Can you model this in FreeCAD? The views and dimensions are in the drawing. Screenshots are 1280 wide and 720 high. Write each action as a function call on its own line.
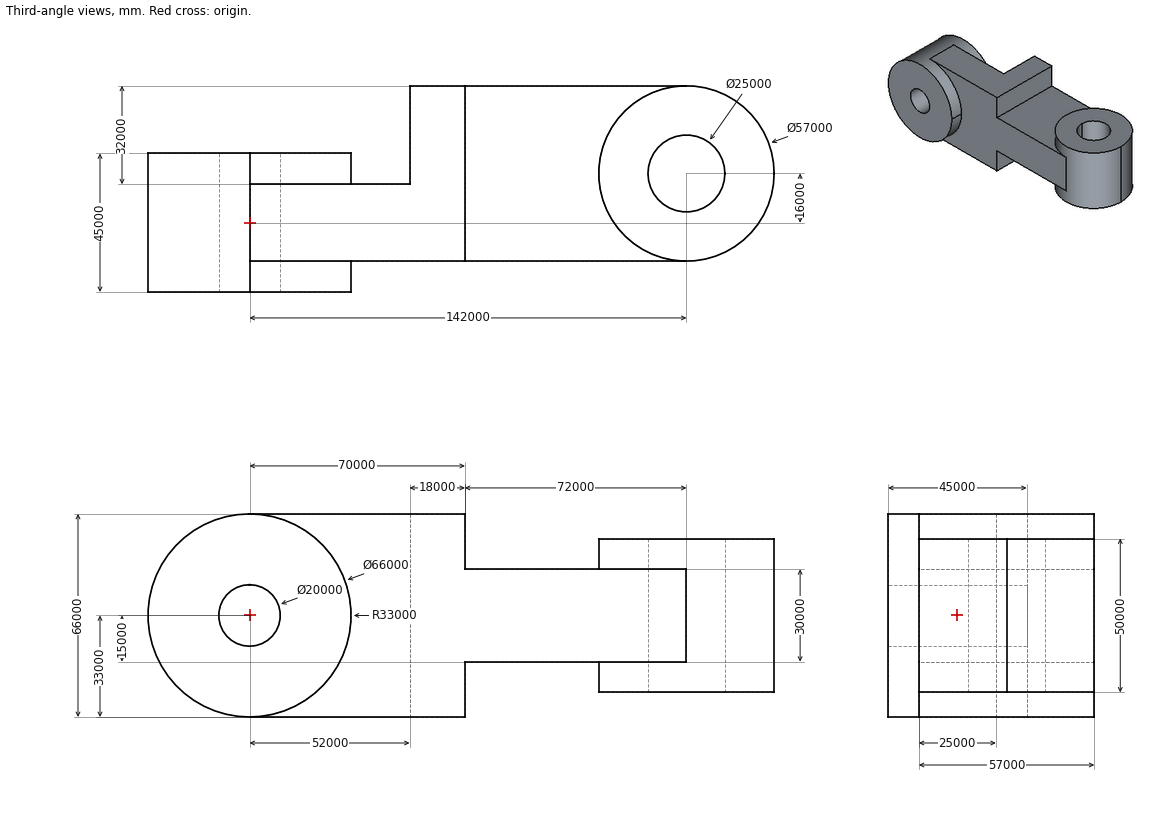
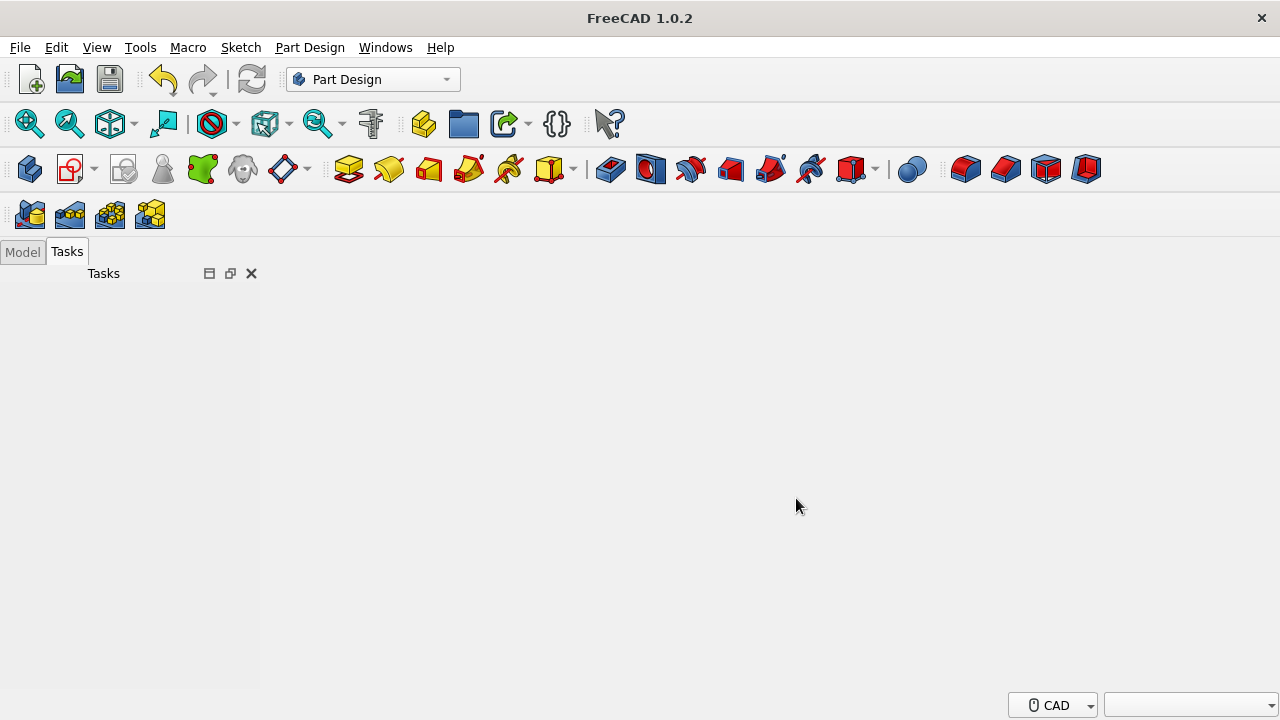
key(ctrl+n)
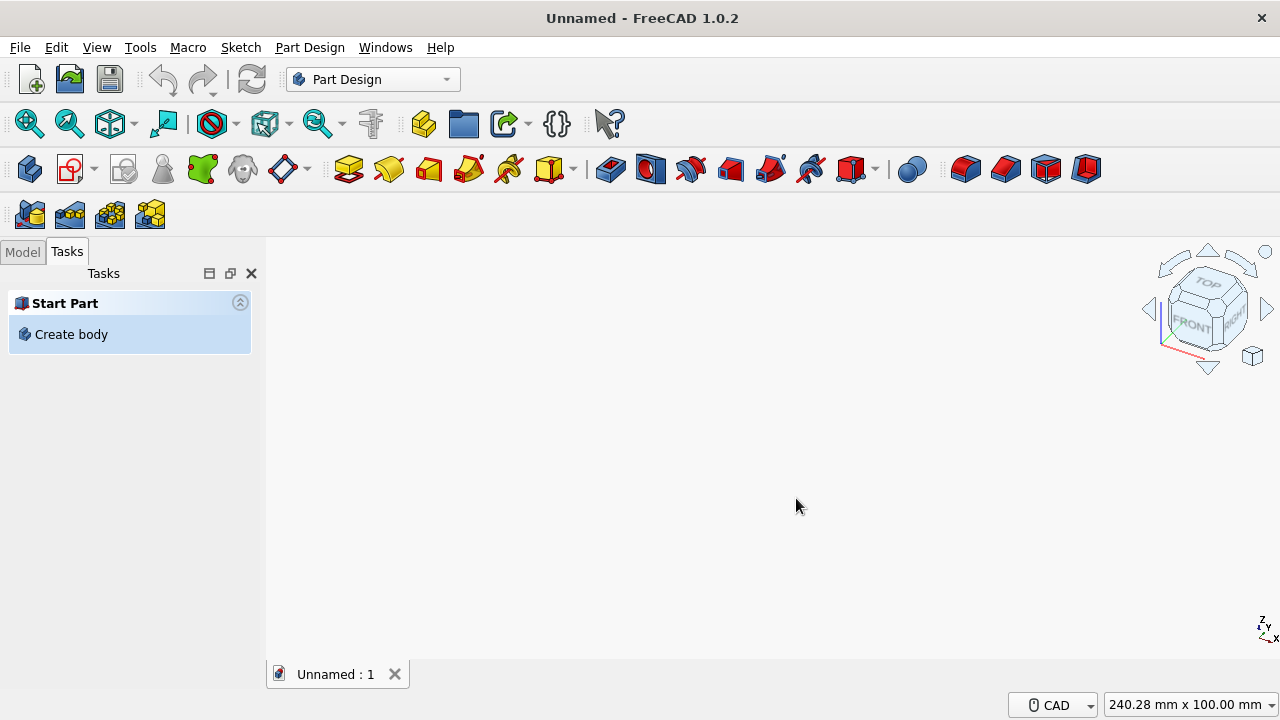
click(70, 170)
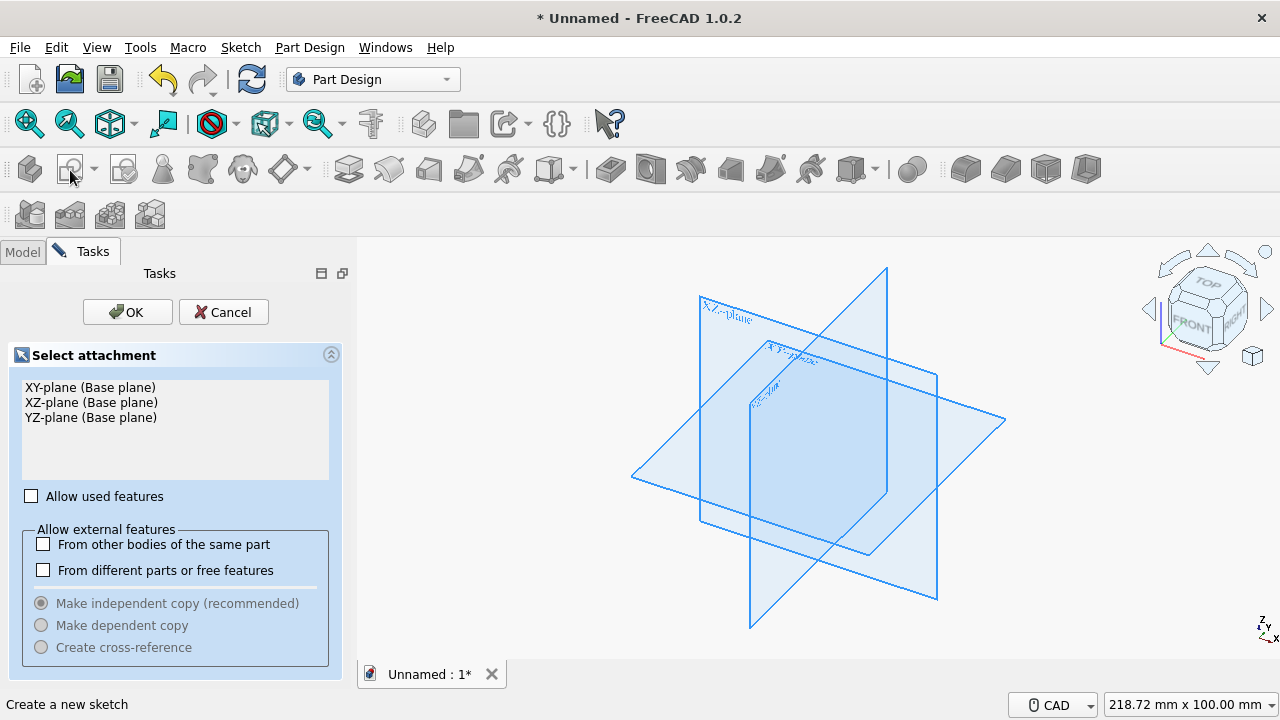
click(82, 402)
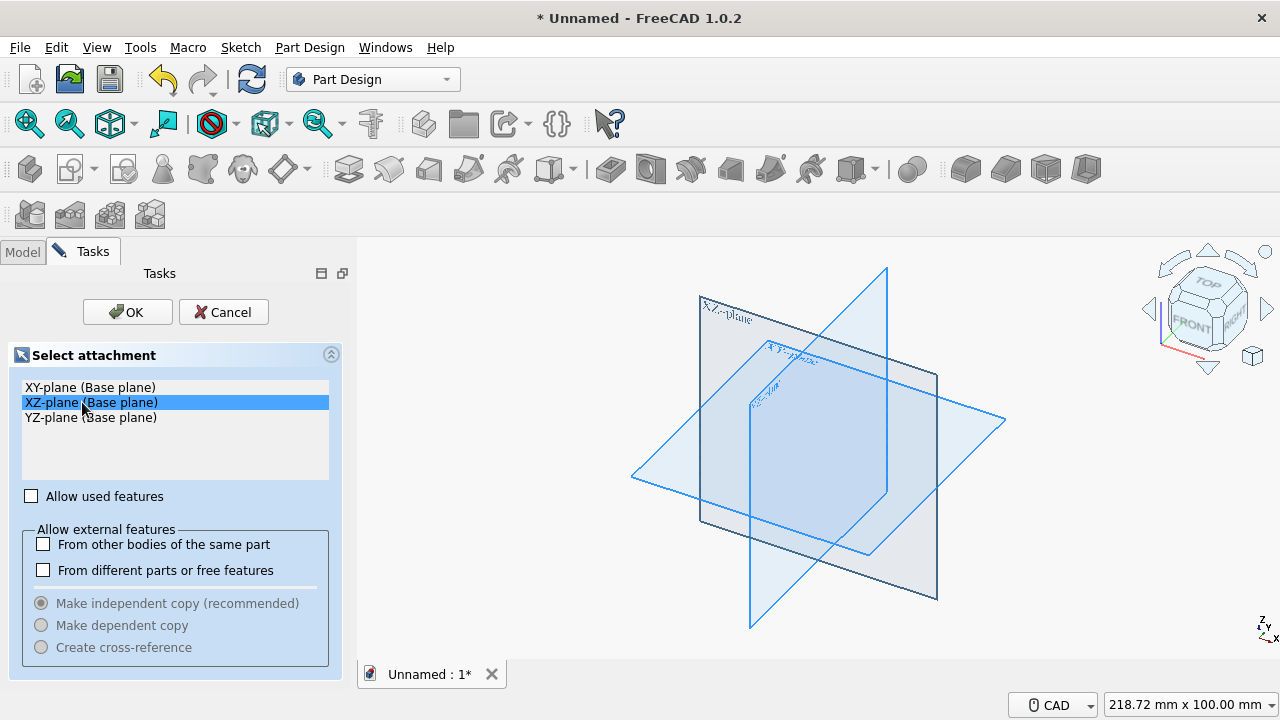
click(128, 312)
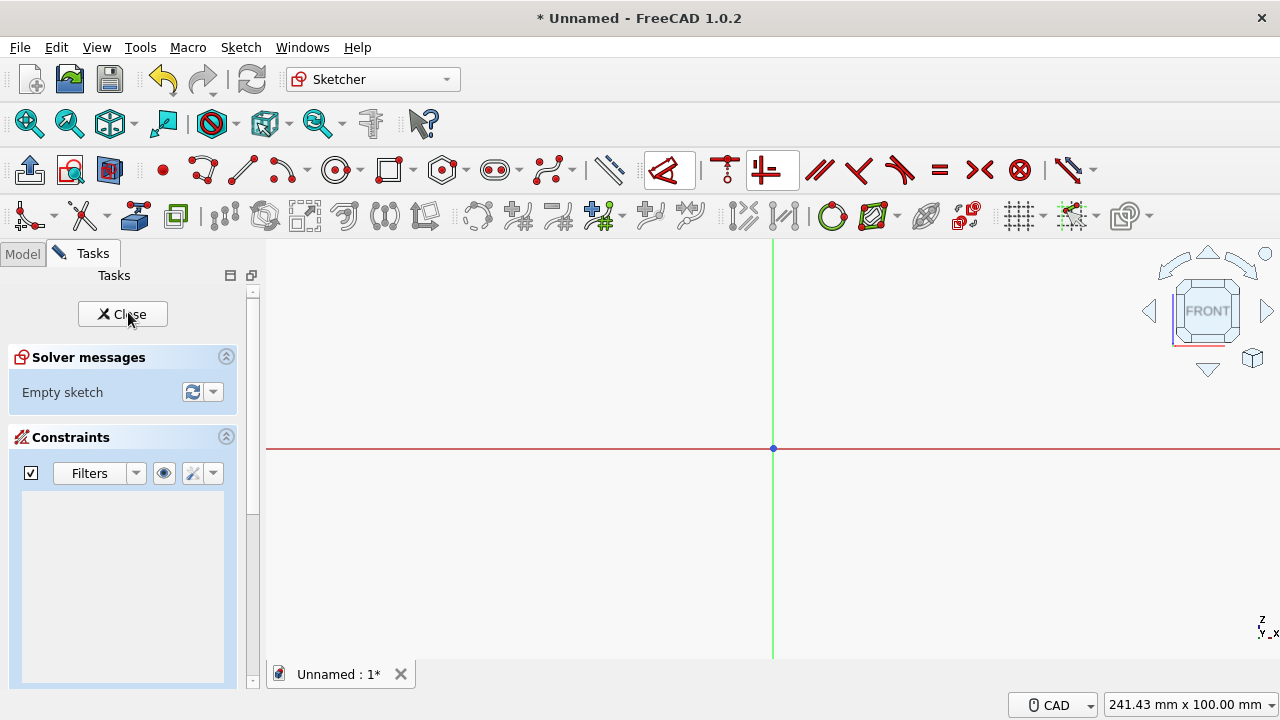
scroll(704, 449, down, 15)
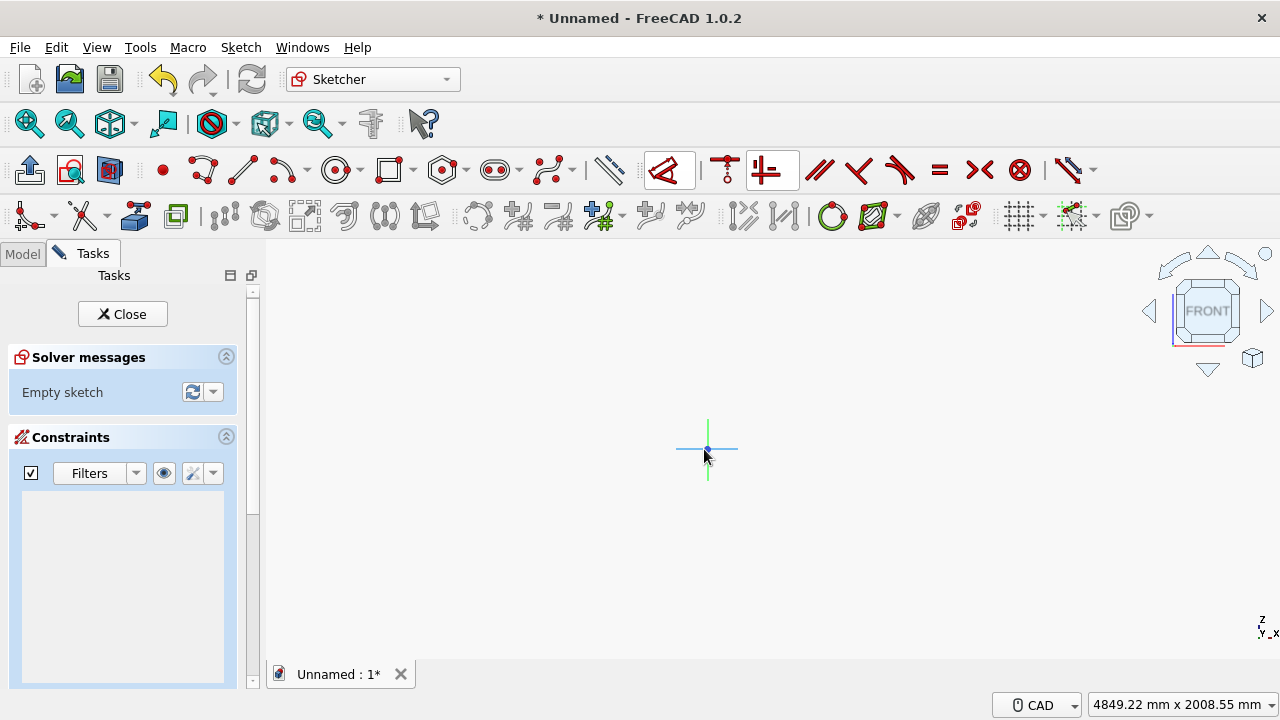
scroll(704, 449, down, 15)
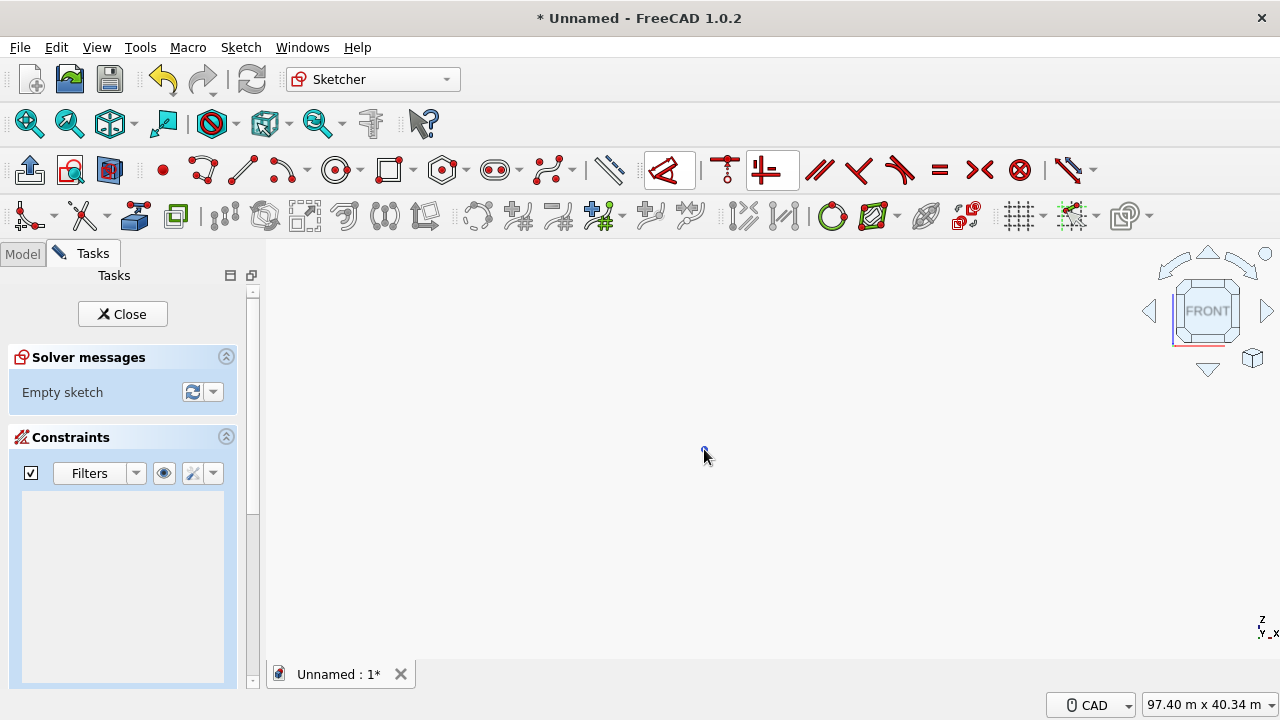
scroll(704, 449, down, 5)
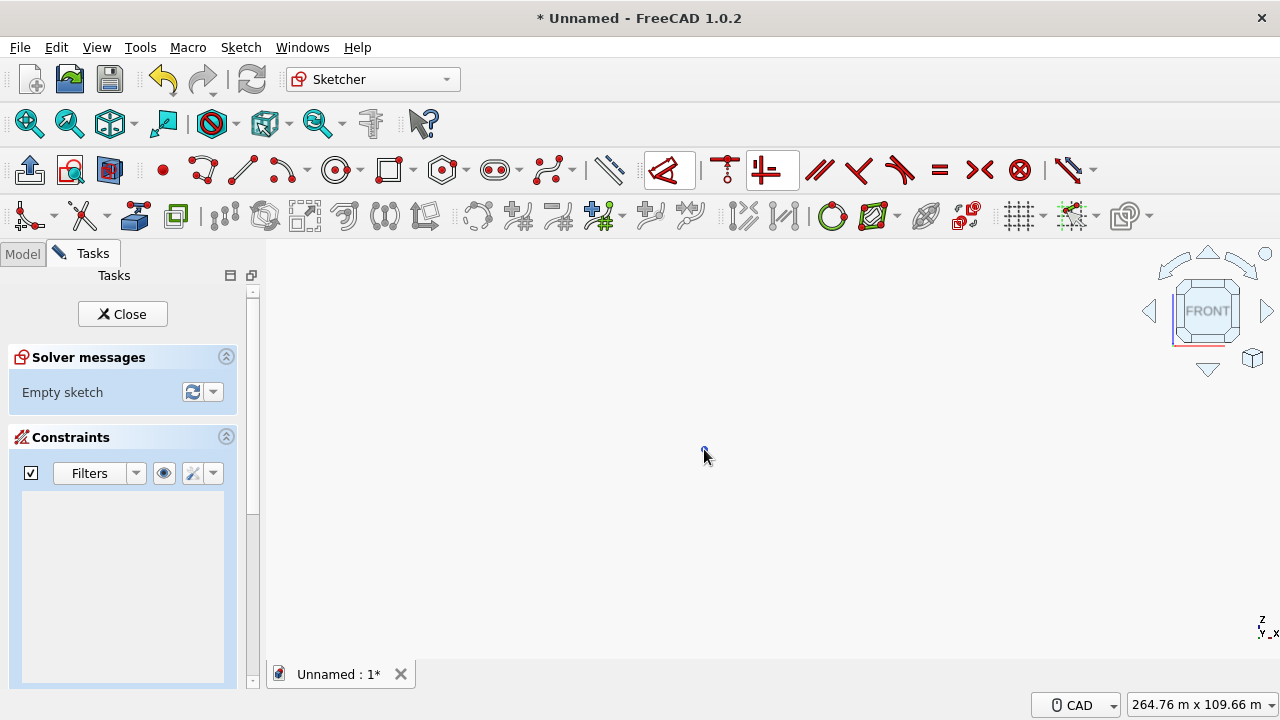
key(g)
key(c)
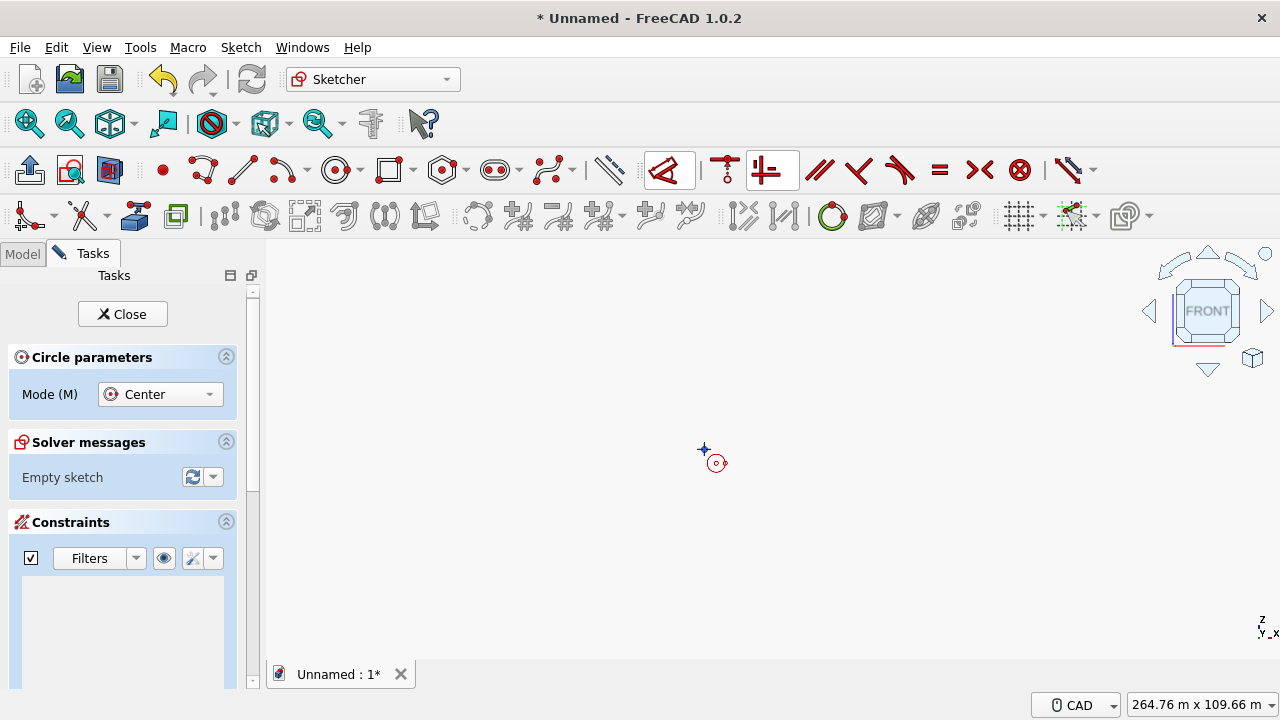
click(704, 450)
click(794, 360)
key(Escape)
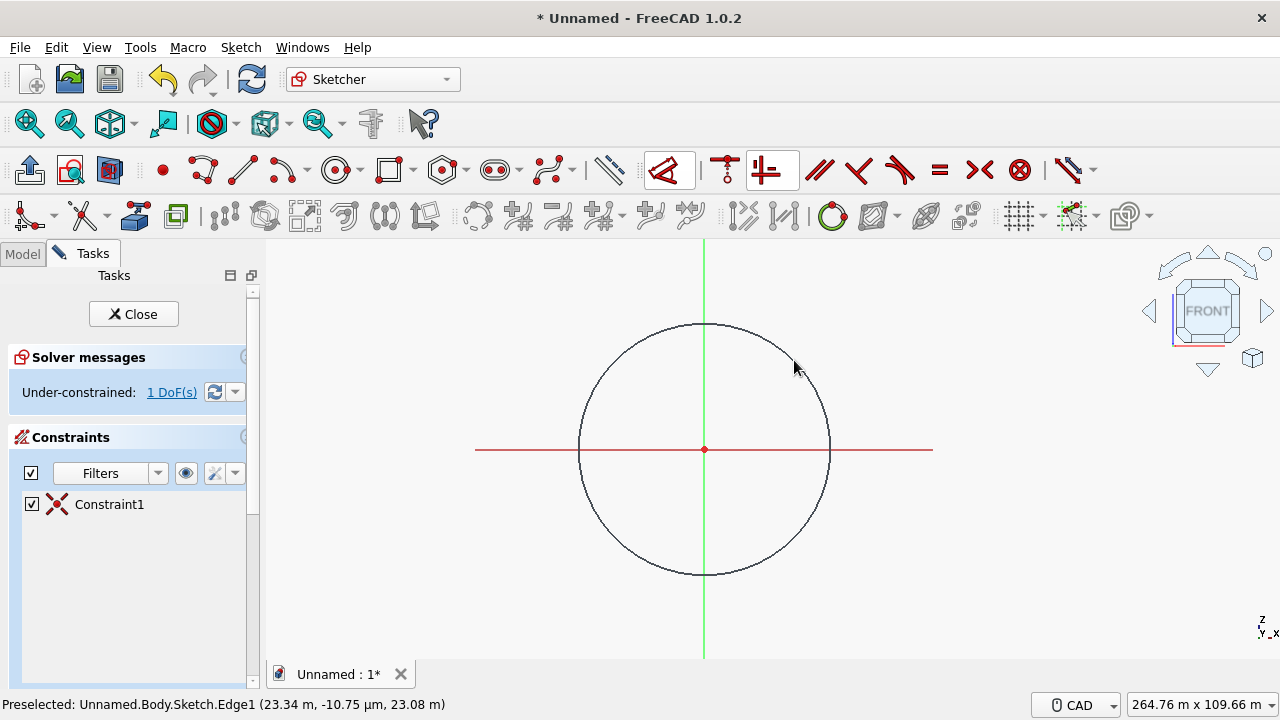
key(d)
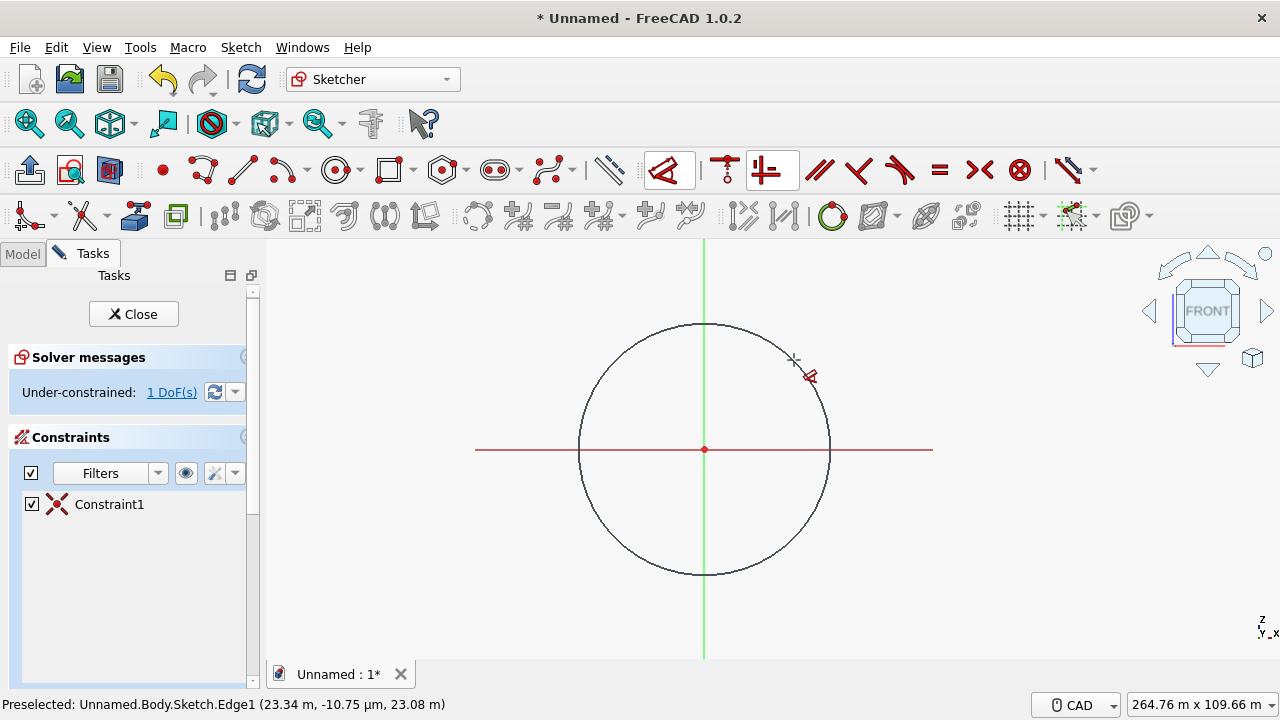
click(793, 360)
click(816, 337)